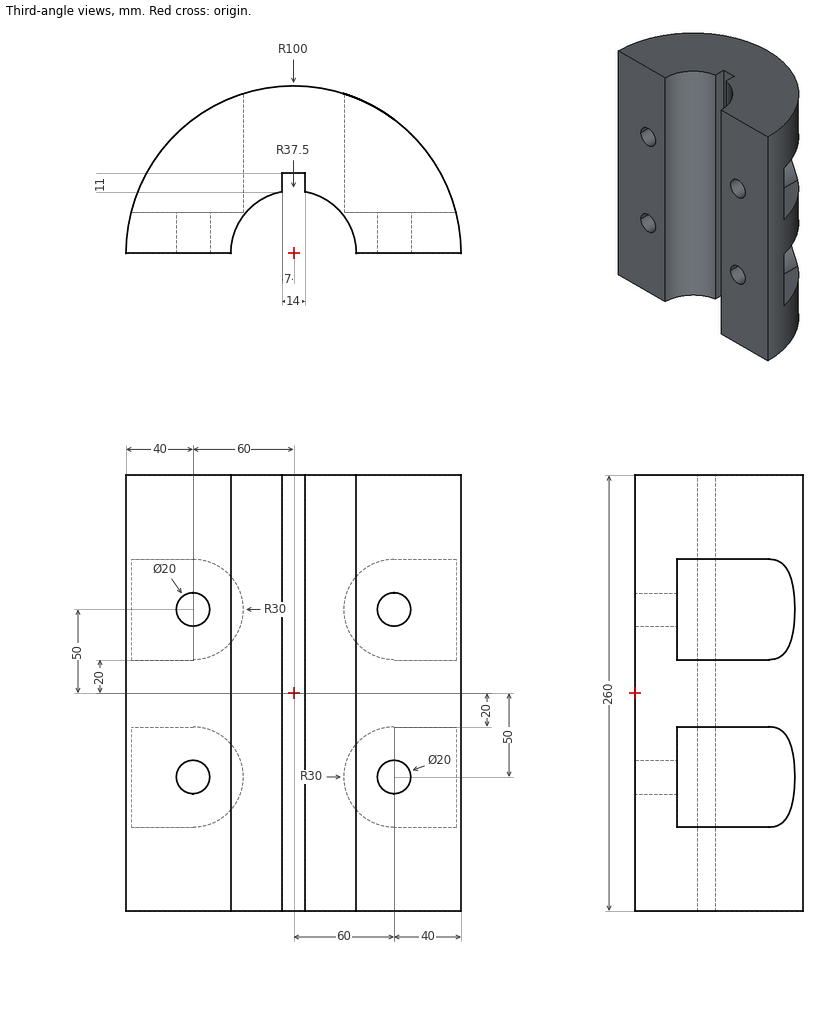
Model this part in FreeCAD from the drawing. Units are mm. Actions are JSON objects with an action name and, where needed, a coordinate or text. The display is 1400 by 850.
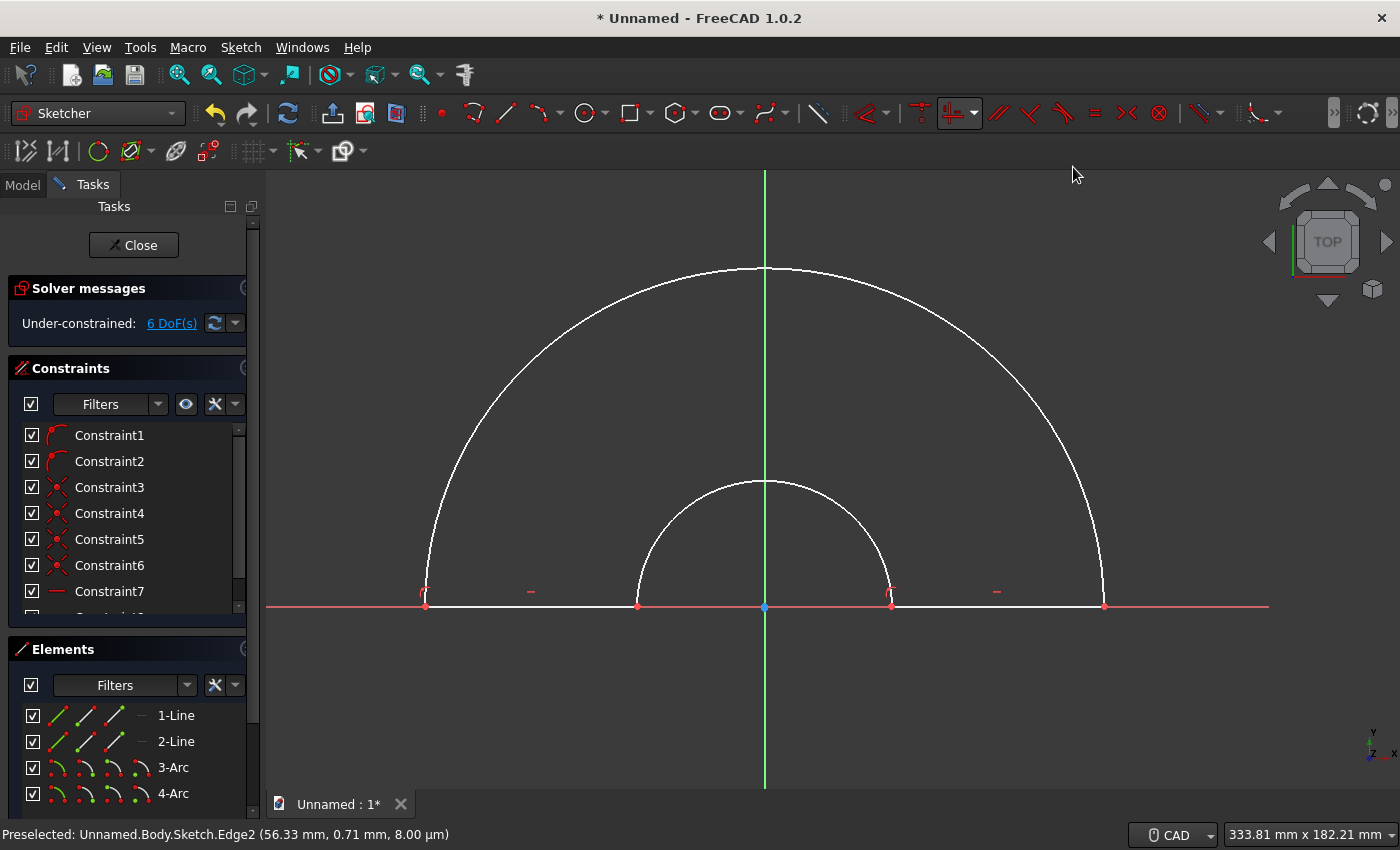
{"action": "left_click", "coordinate": [839, 505]}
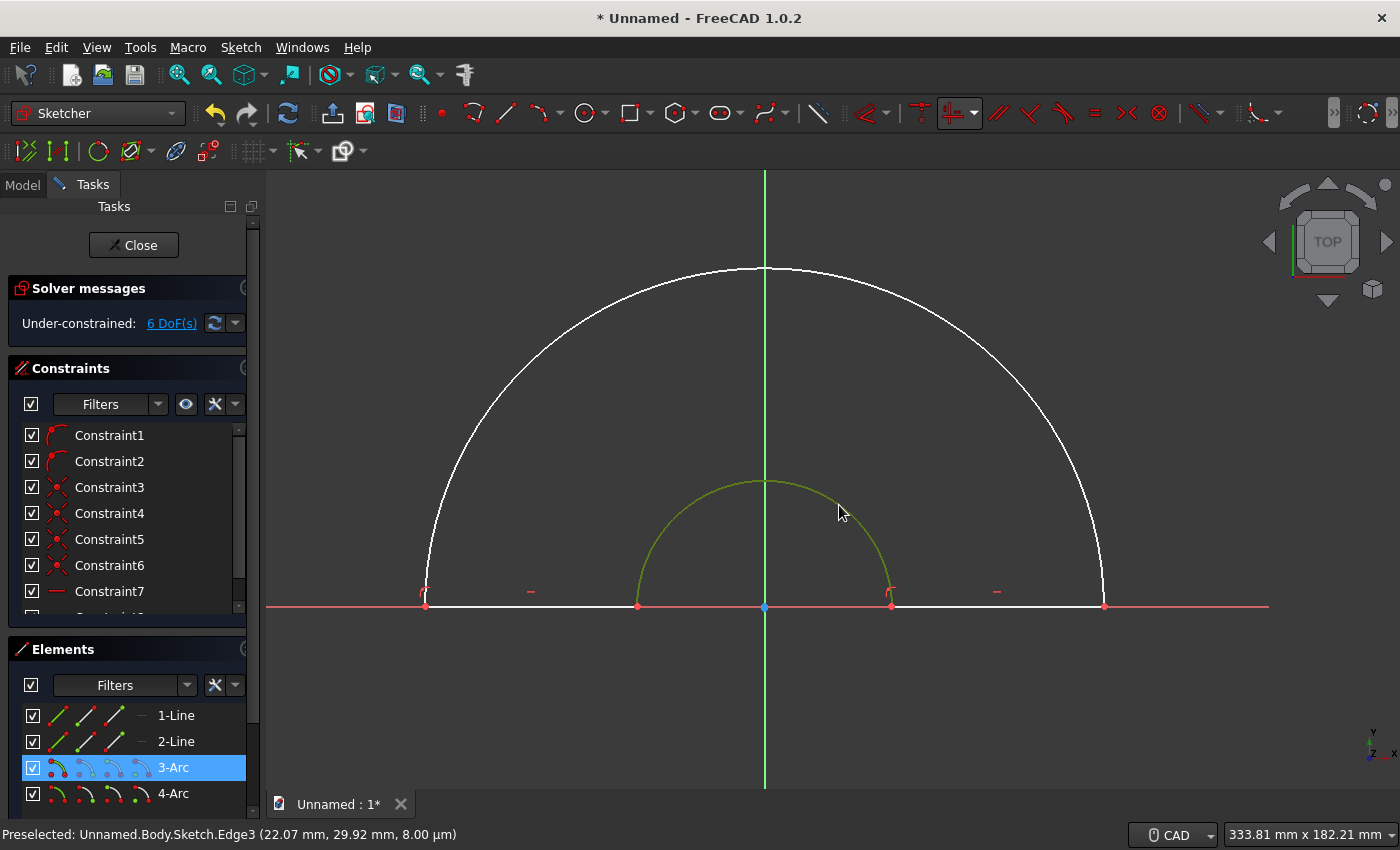
{"action": "left_click", "coordinate": [964, 333]}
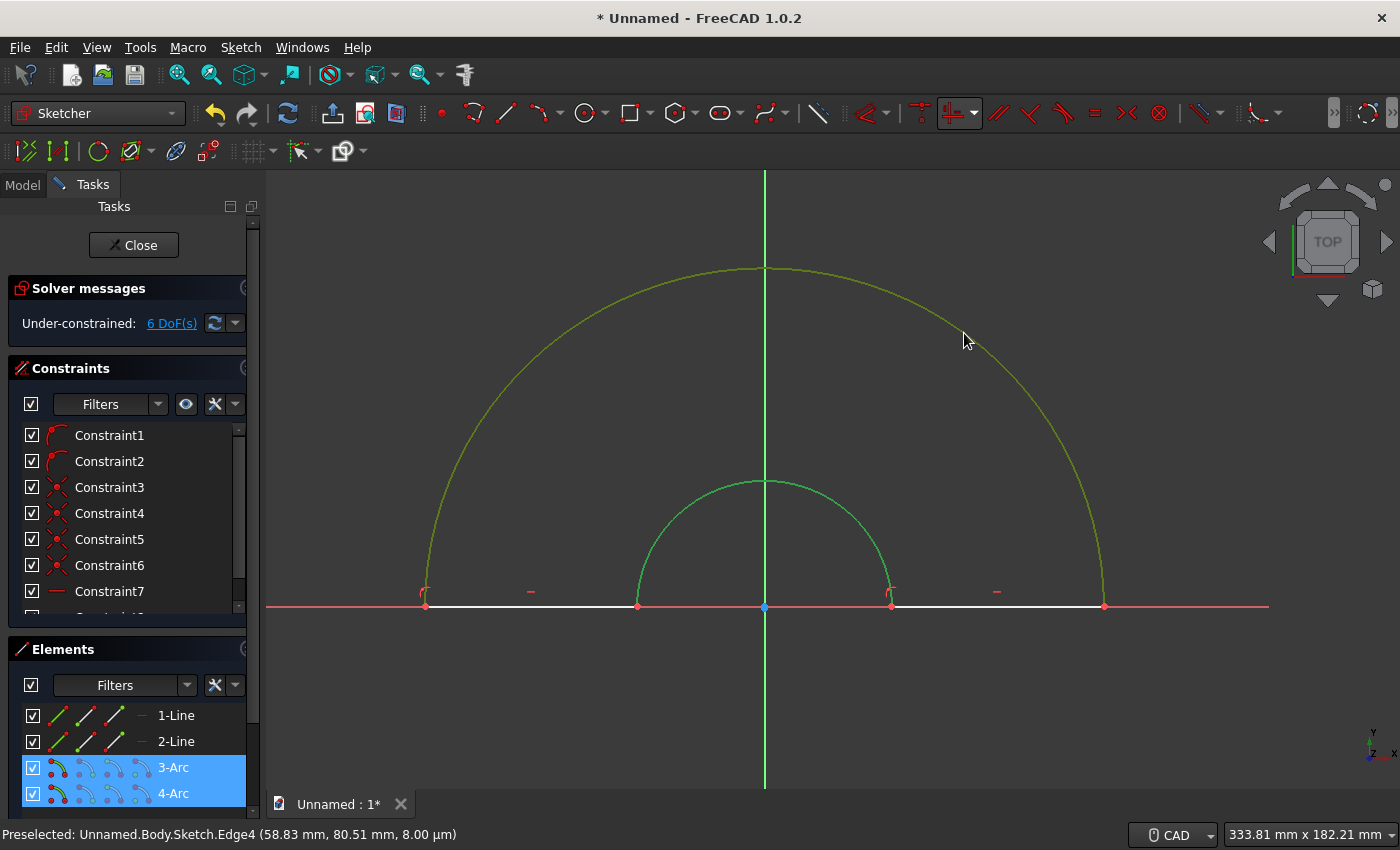
{"action": "left_click", "coordinate": [920, 114]}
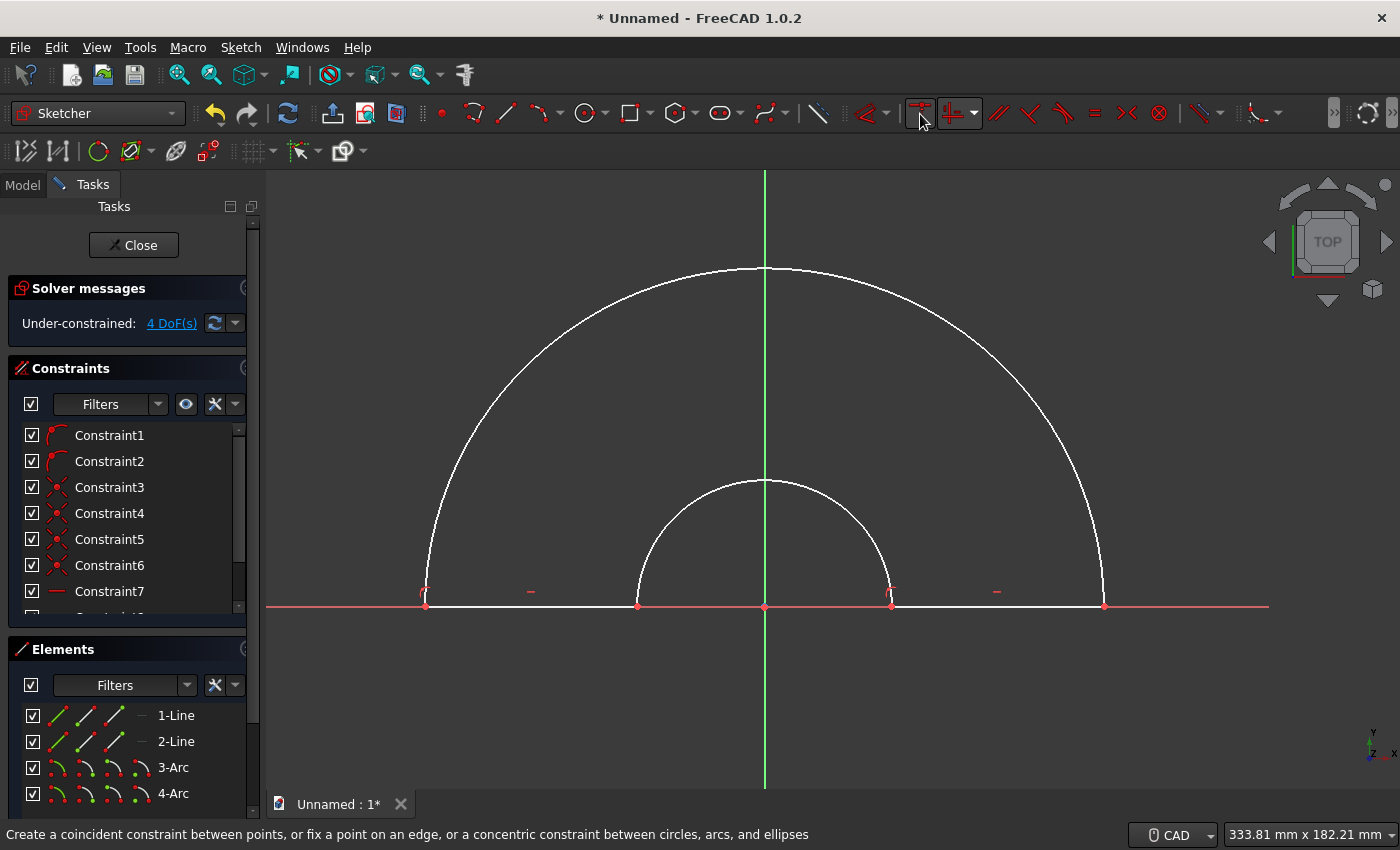
{"action": "left_click_drag", "start_coordinate": [755, 597], "coordinate": [775, 618]}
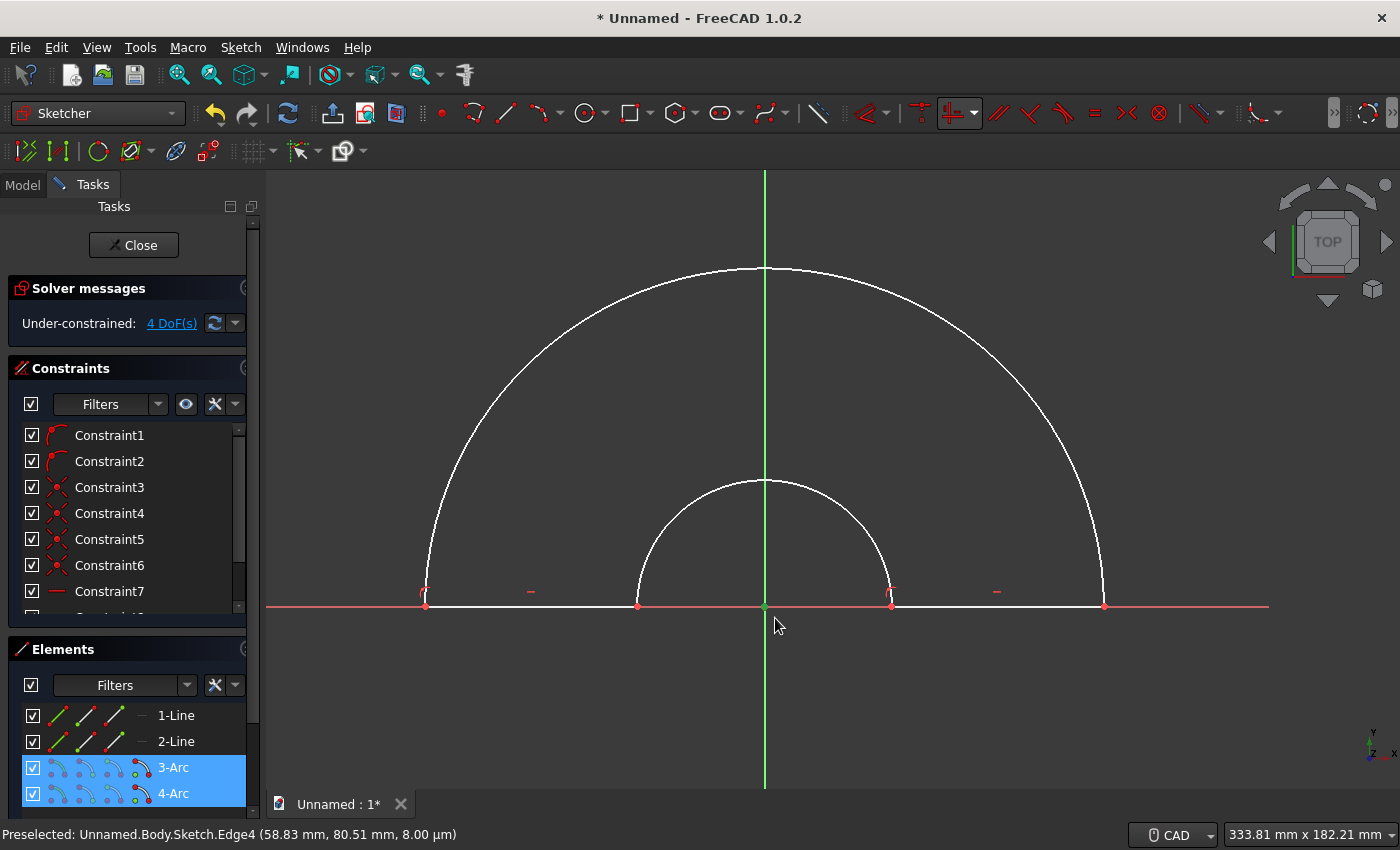
{"action": "left_click", "coordinate": [920, 114]}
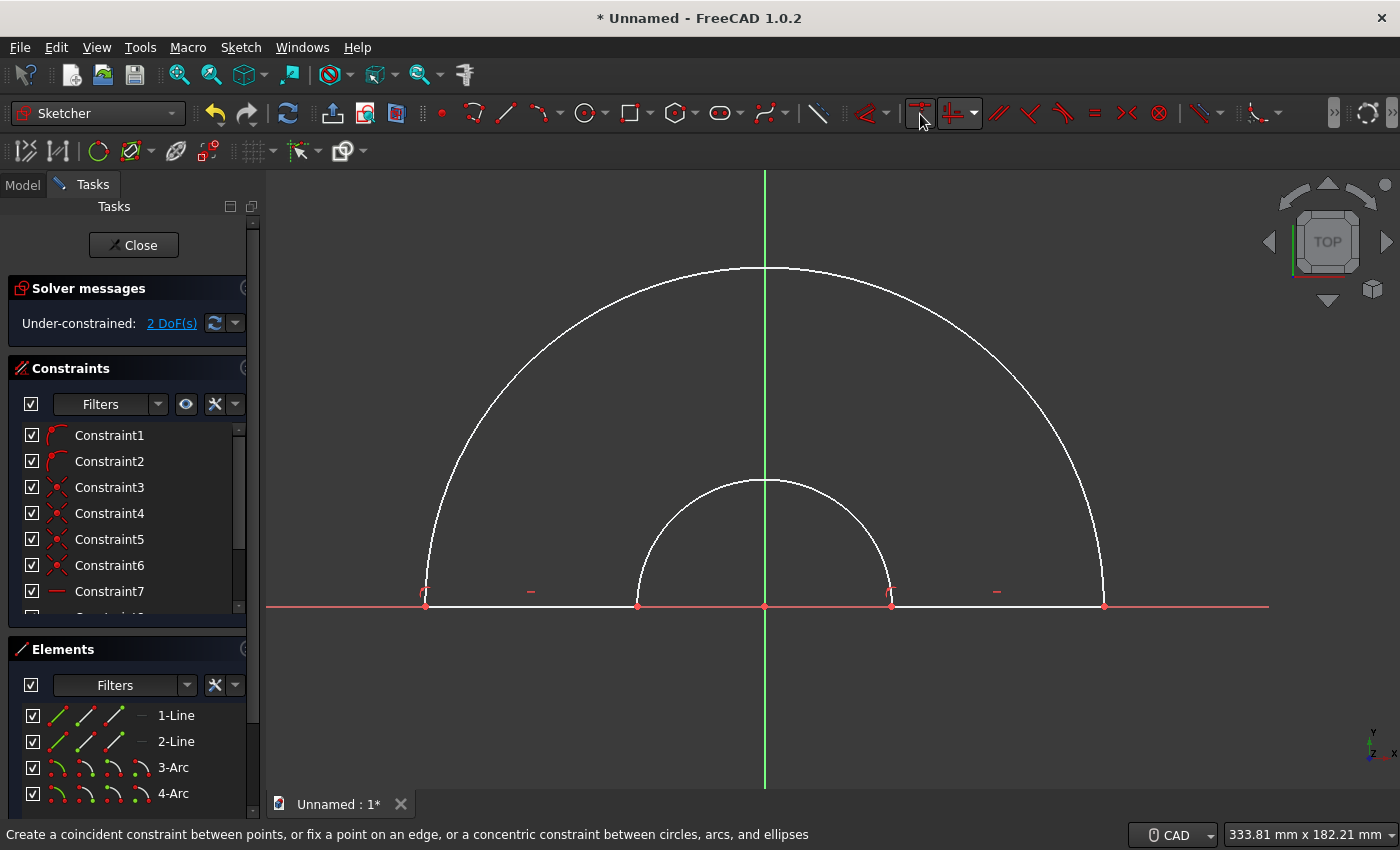
{"action": "left_click", "coordinate": [866, 114]}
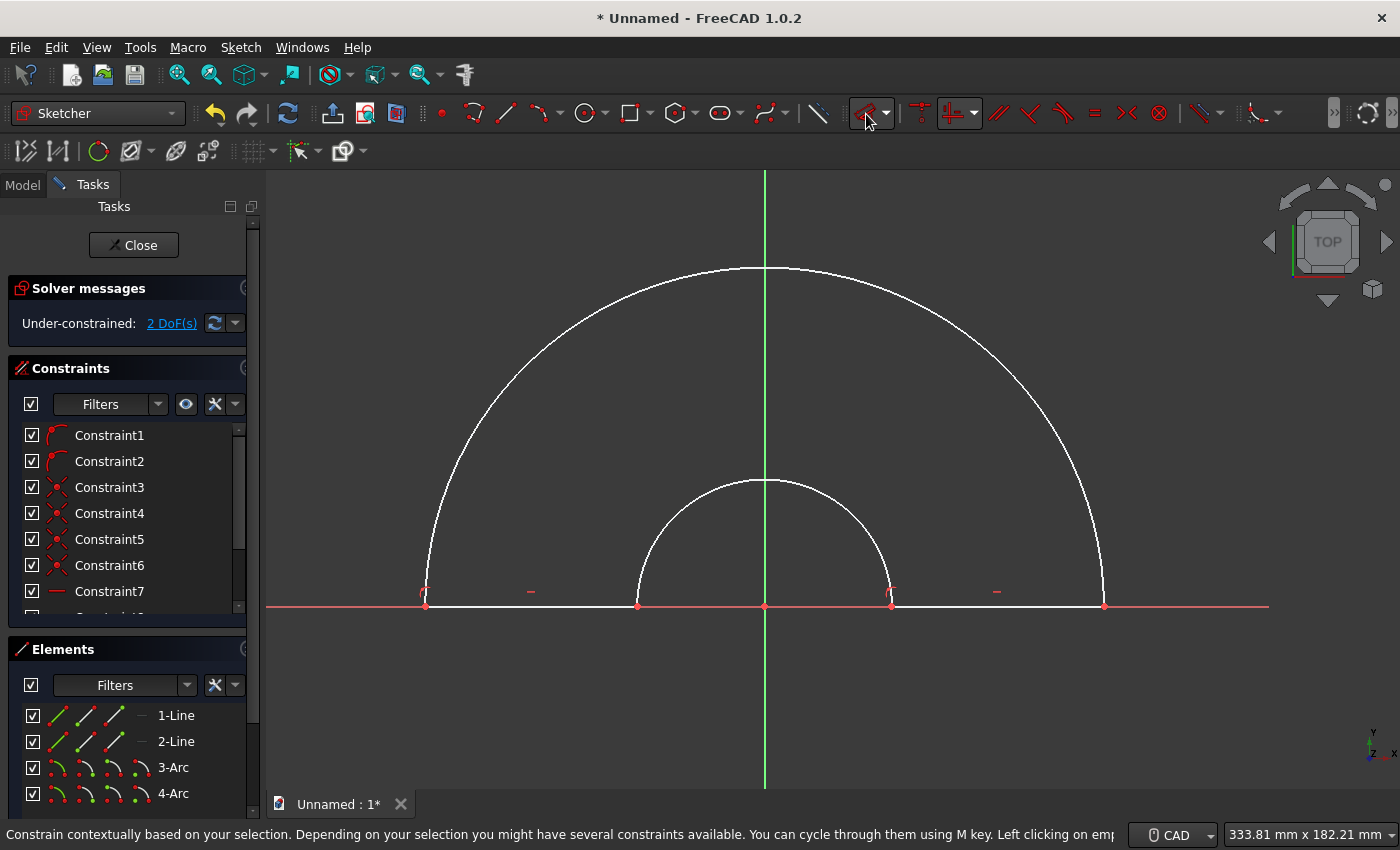
{"action": "left_click", "coordinate": [839, 504]}
{"action": "left_click", "coordinate": [858, 478]}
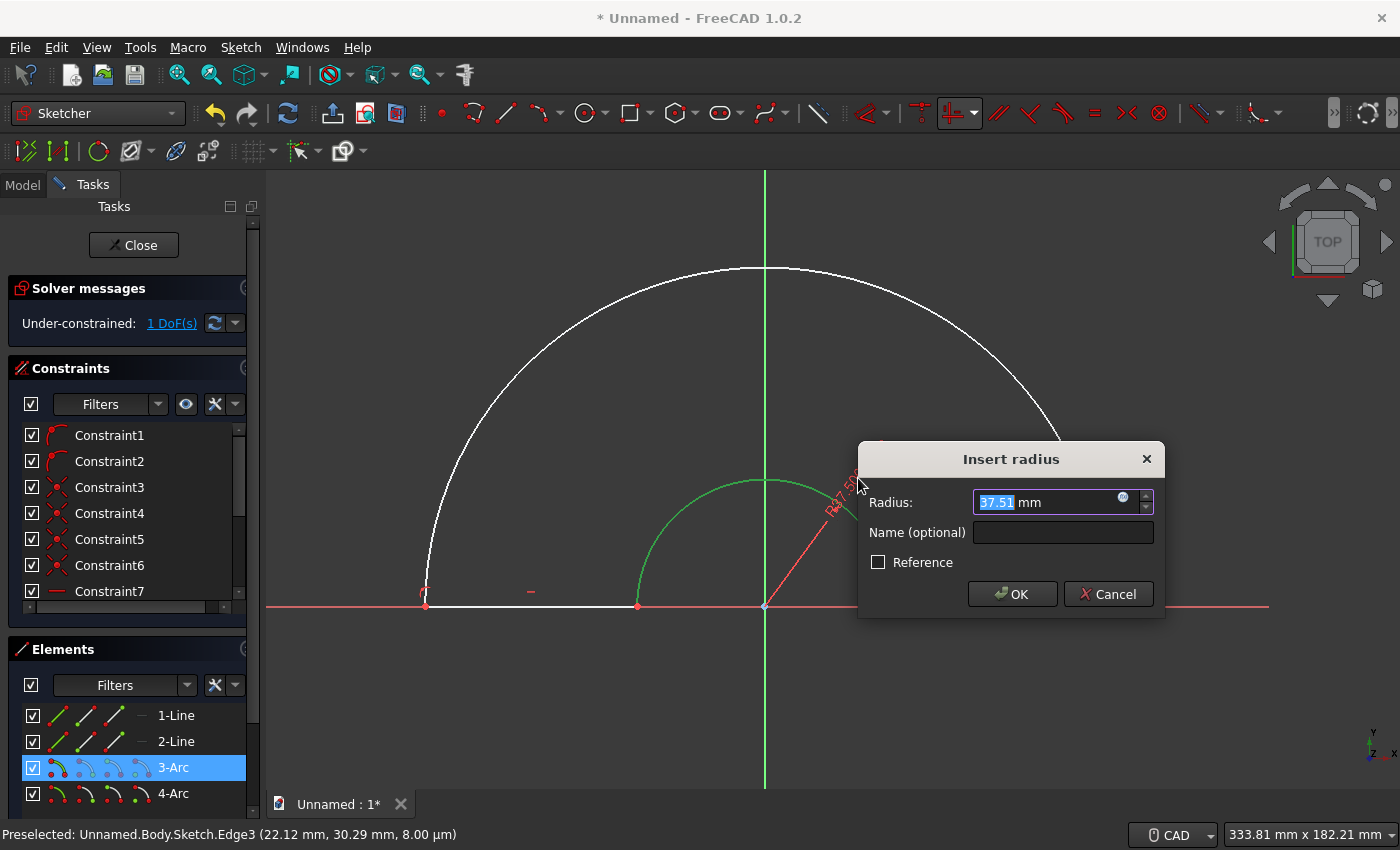
{"action": "type", "text": "37.5"}
{"action": "key", "text": "Return"}